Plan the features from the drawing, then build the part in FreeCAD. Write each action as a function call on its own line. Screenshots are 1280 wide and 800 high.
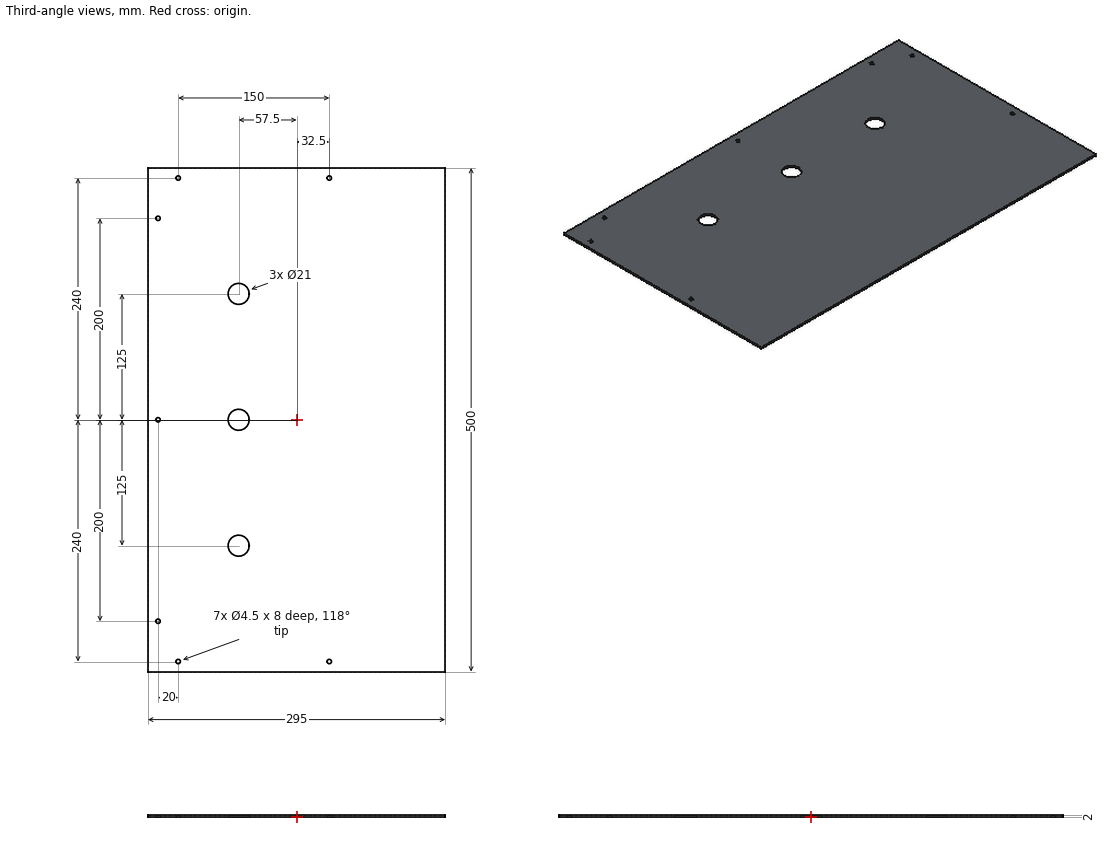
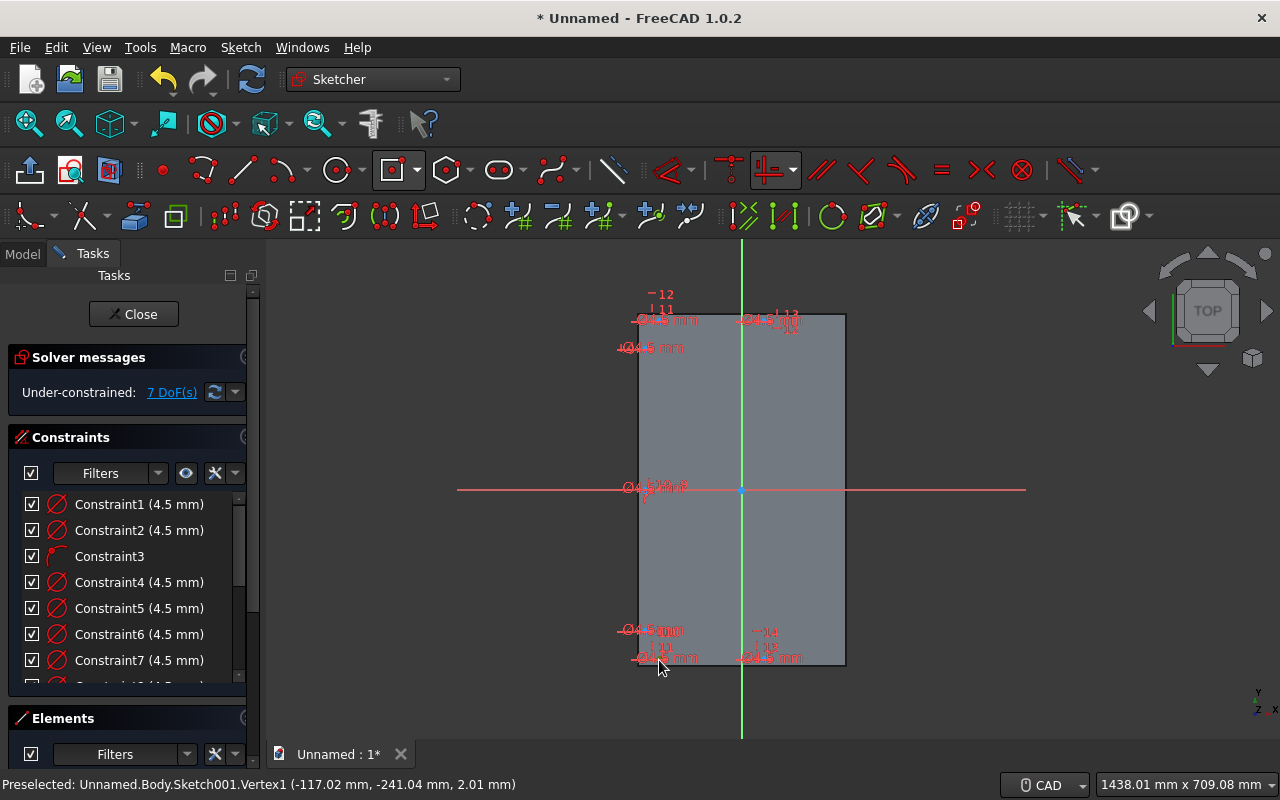
key(i)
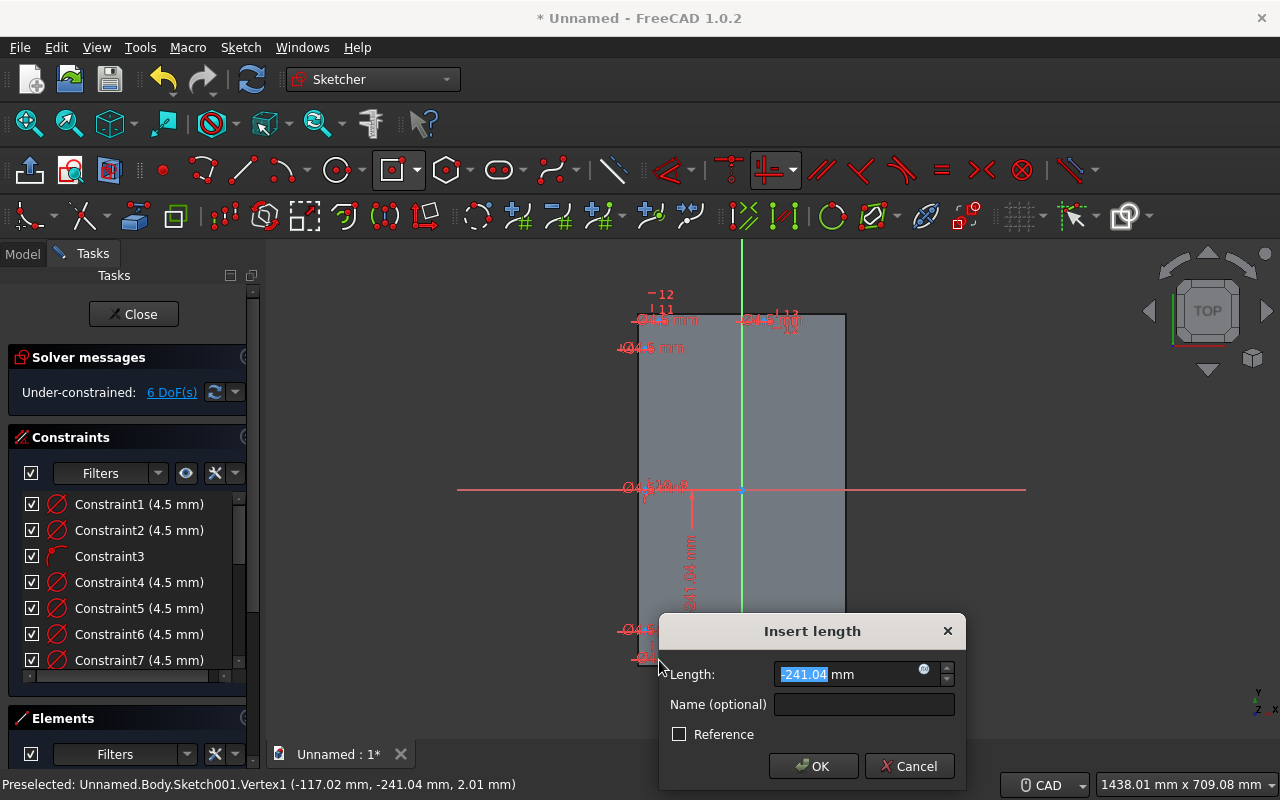
text(-240)
key(Return)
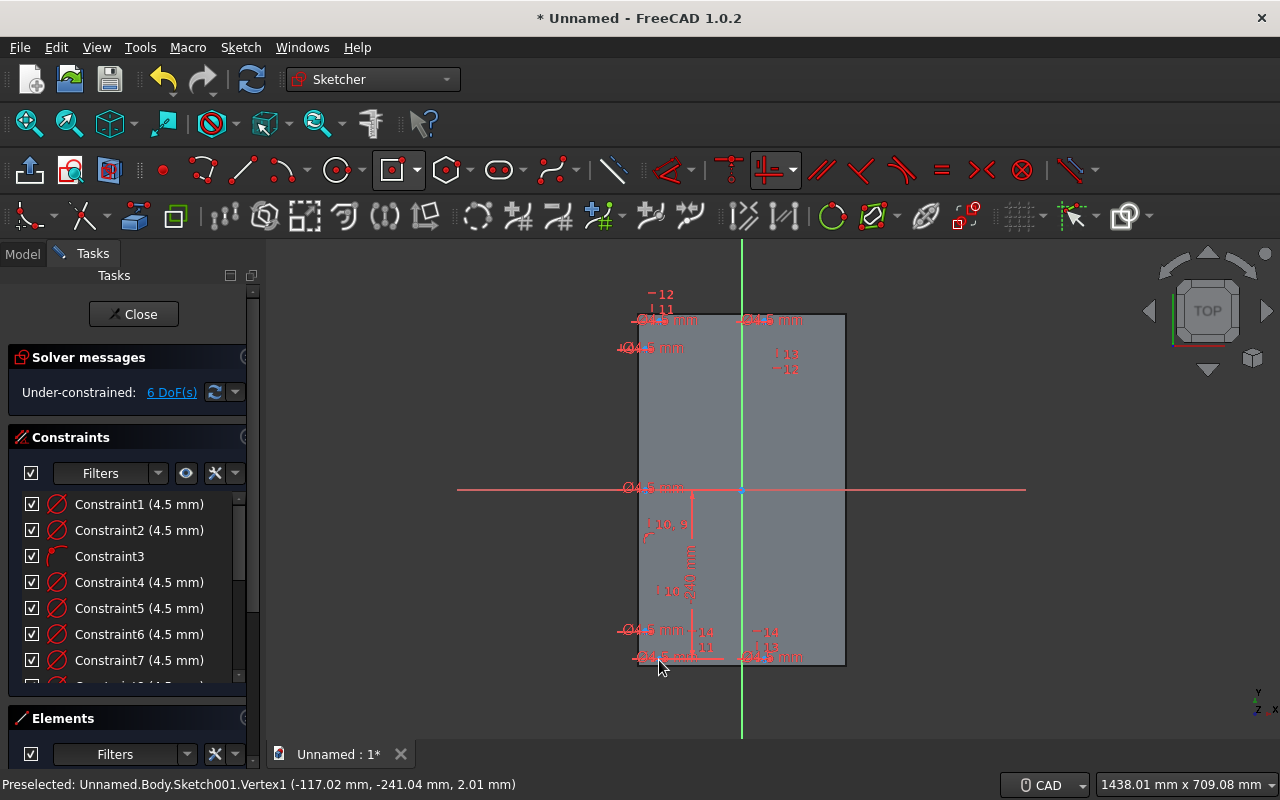
click(645, 350)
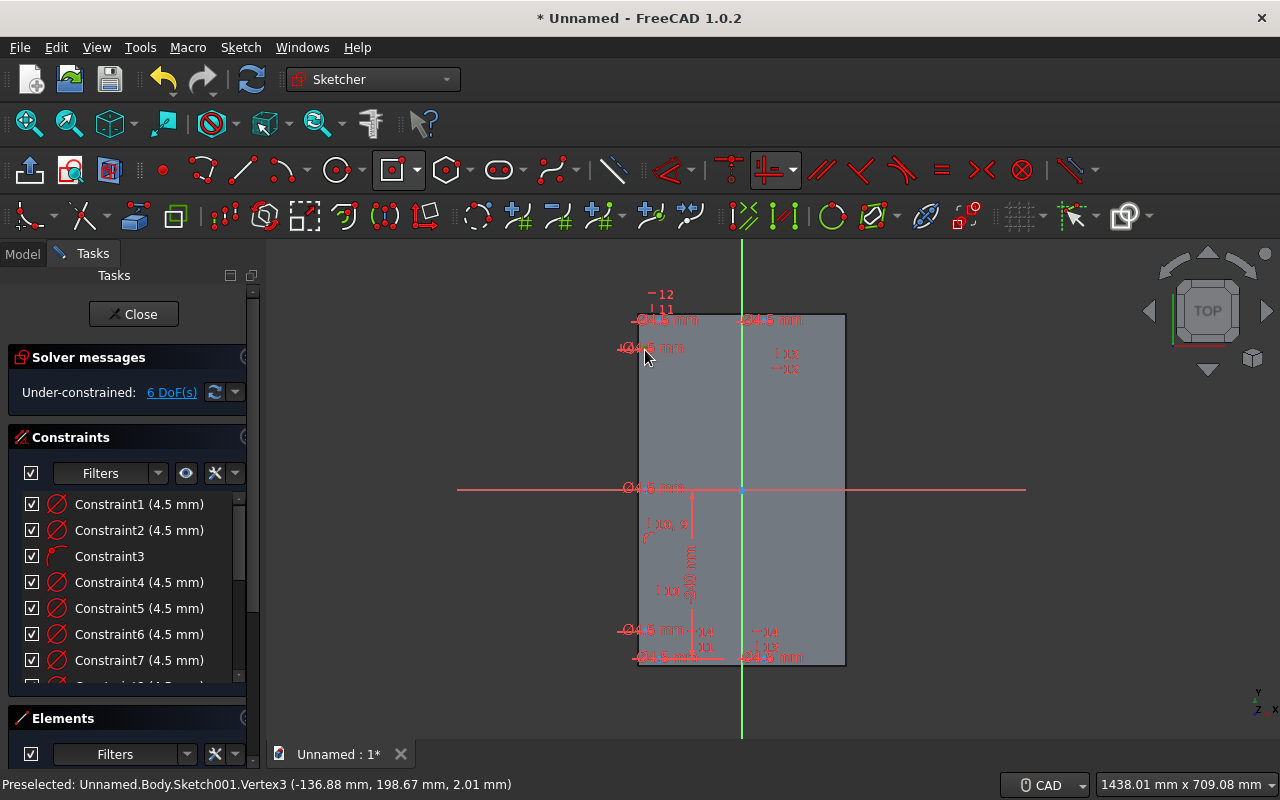
click(694, 170)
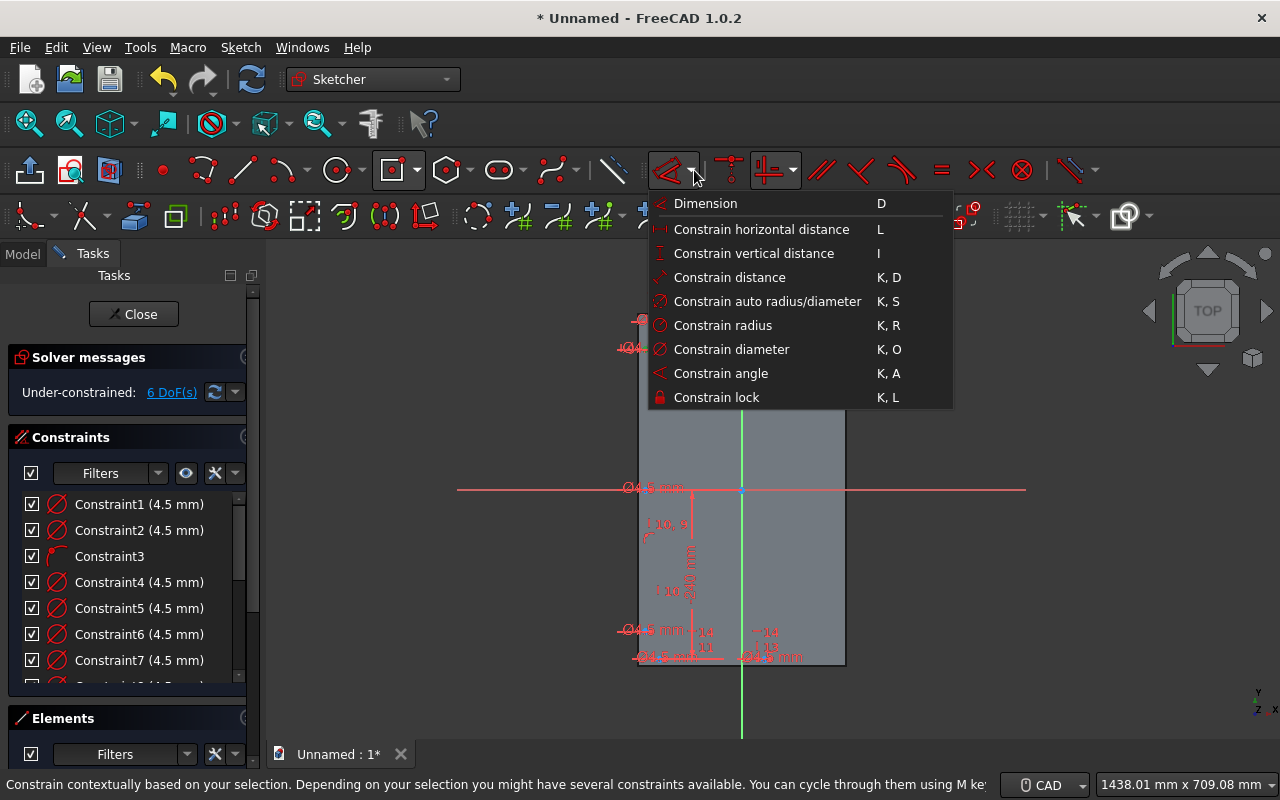
click(801, 253)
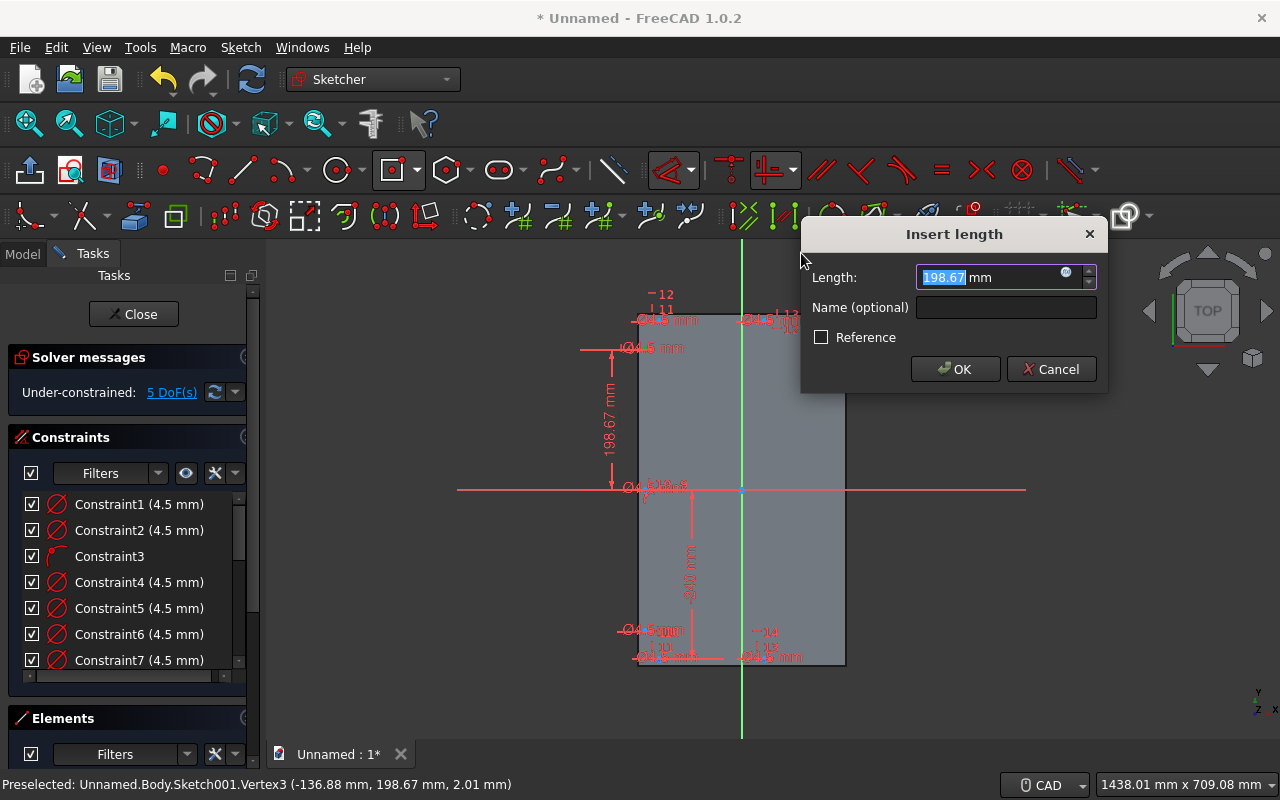
text(200)
key(Return)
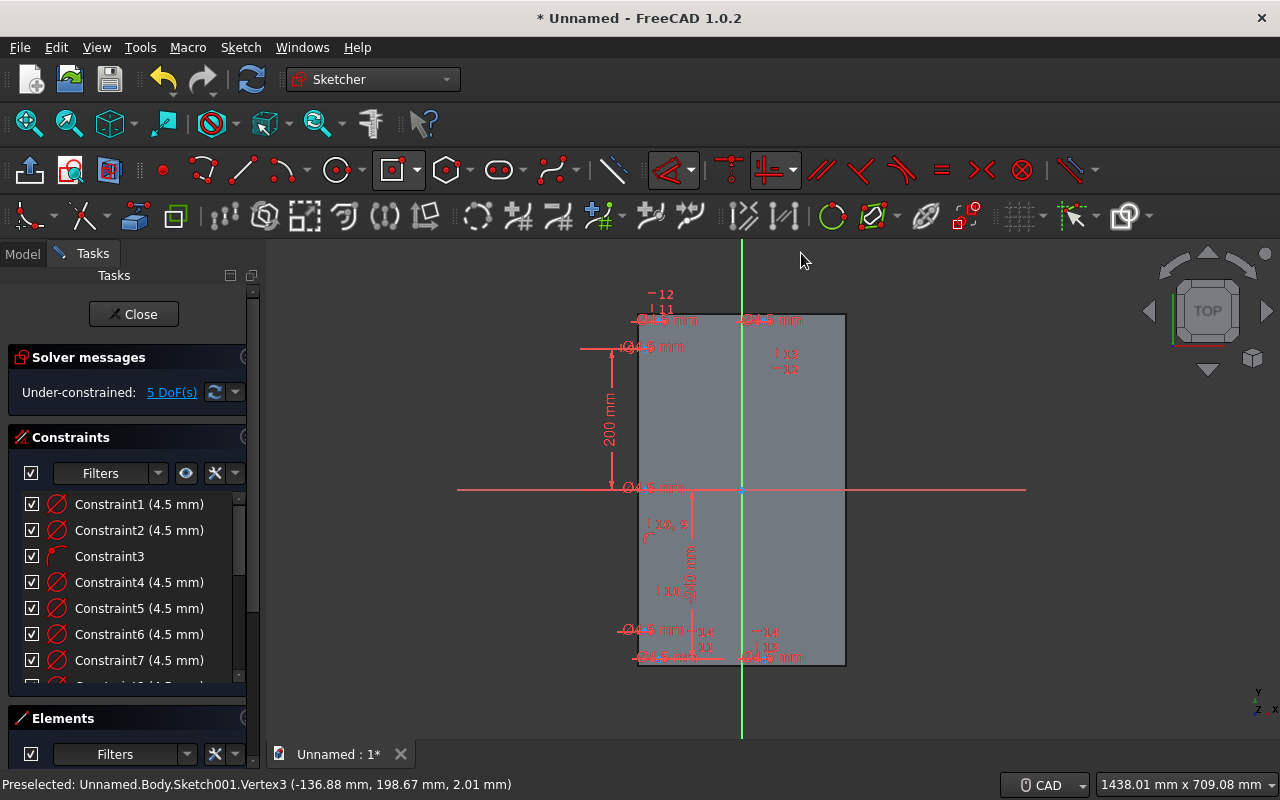
click(645, 632)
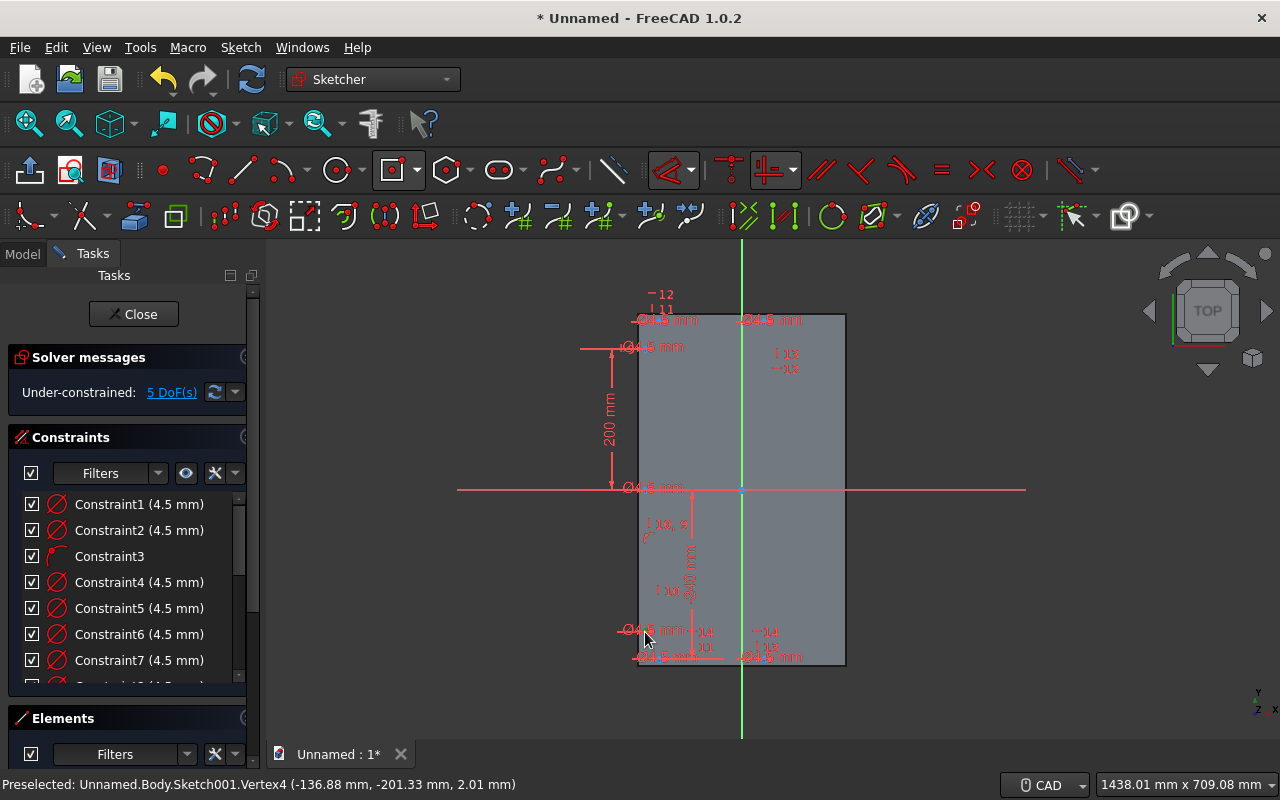
click(694, 170)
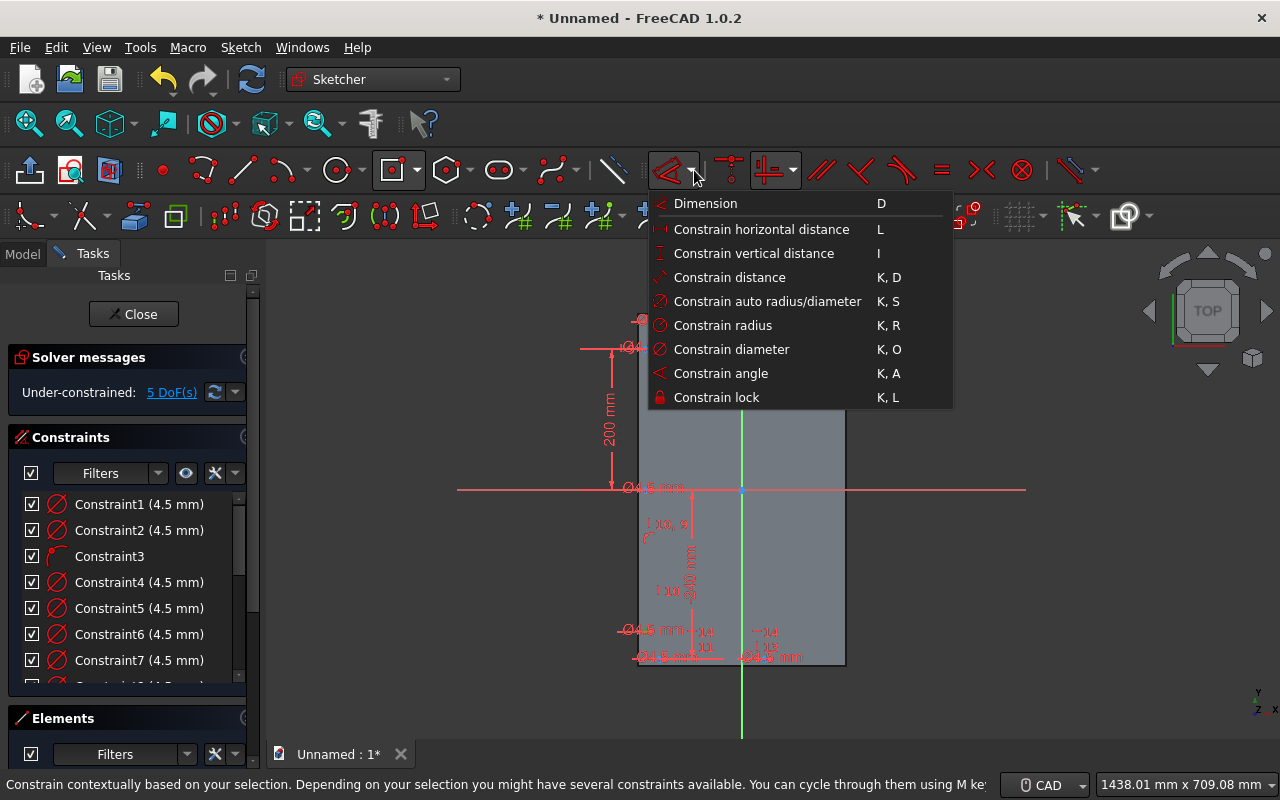
click(801, 253)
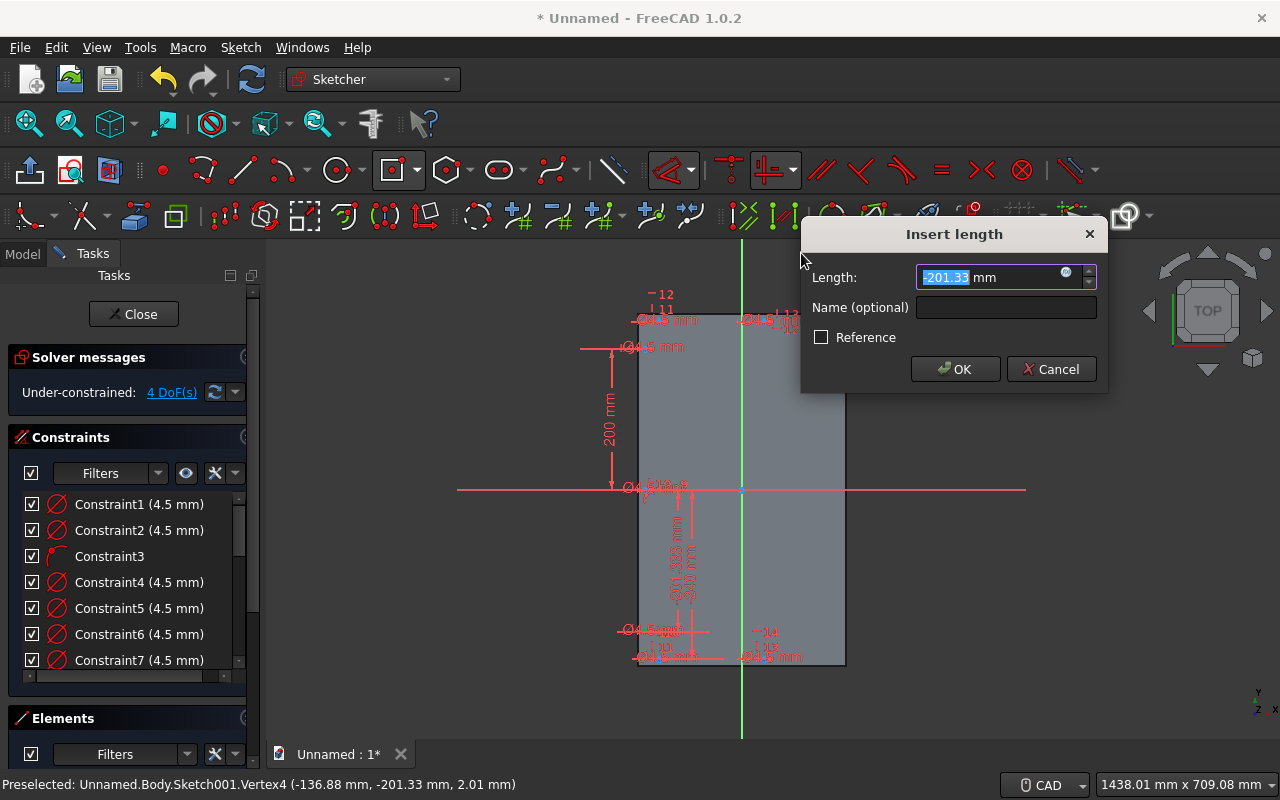
text(-200)
key(Return)